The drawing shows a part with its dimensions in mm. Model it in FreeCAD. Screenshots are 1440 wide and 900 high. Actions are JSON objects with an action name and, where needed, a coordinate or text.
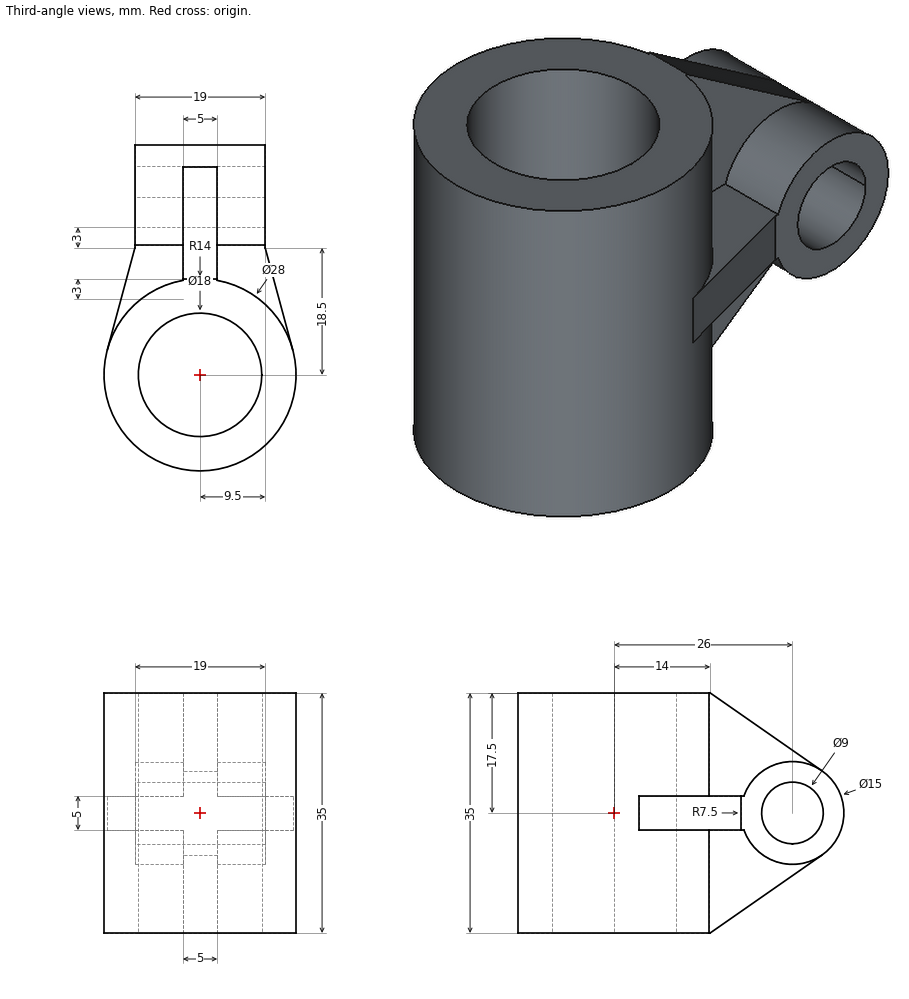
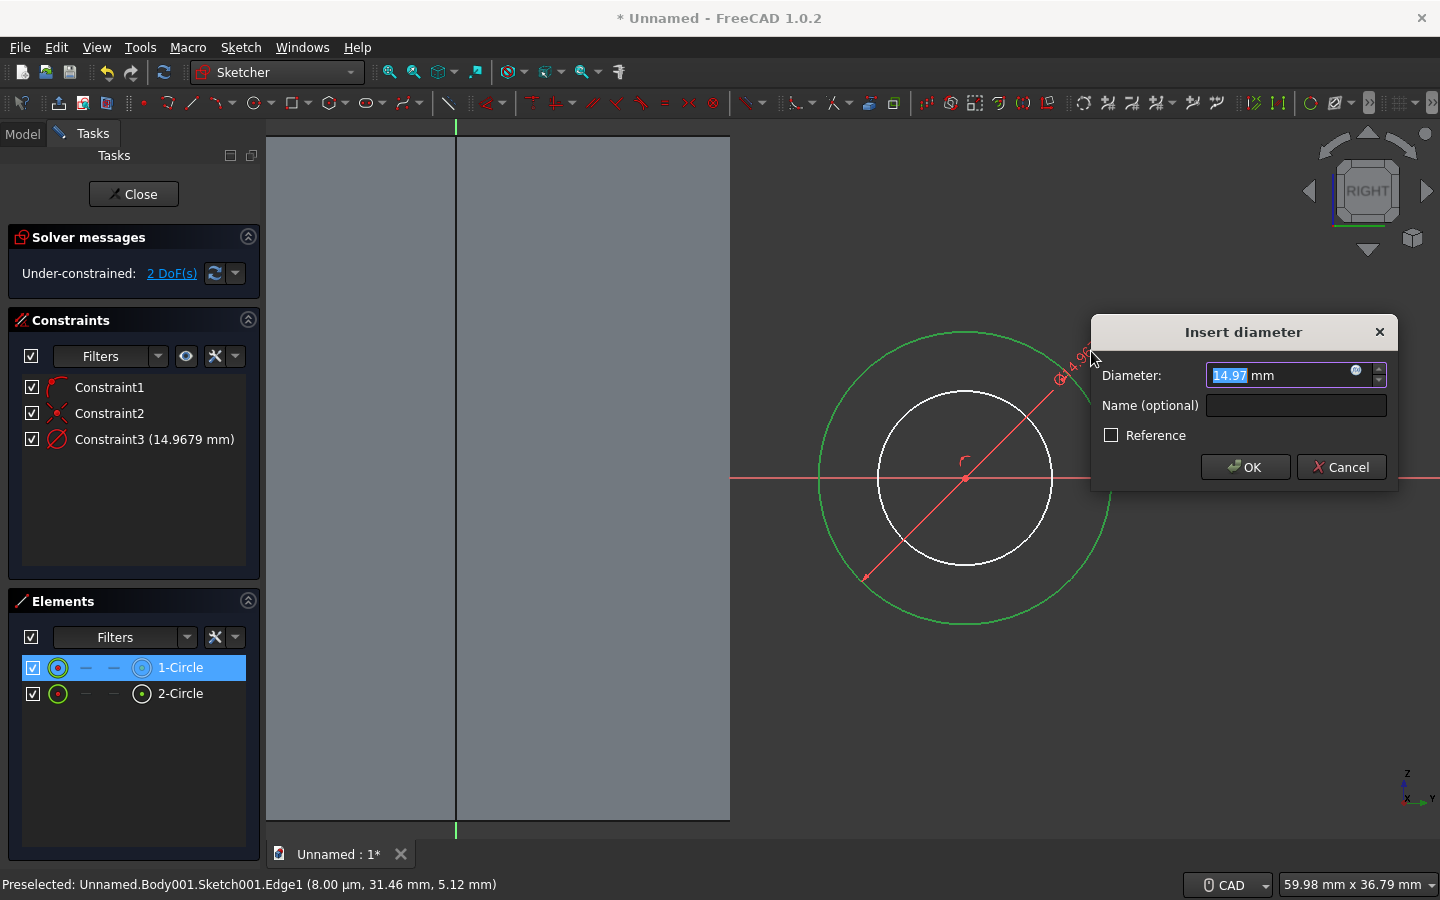
{"action": "type", "text": "15"}
{"action": "key", "text": "Return"}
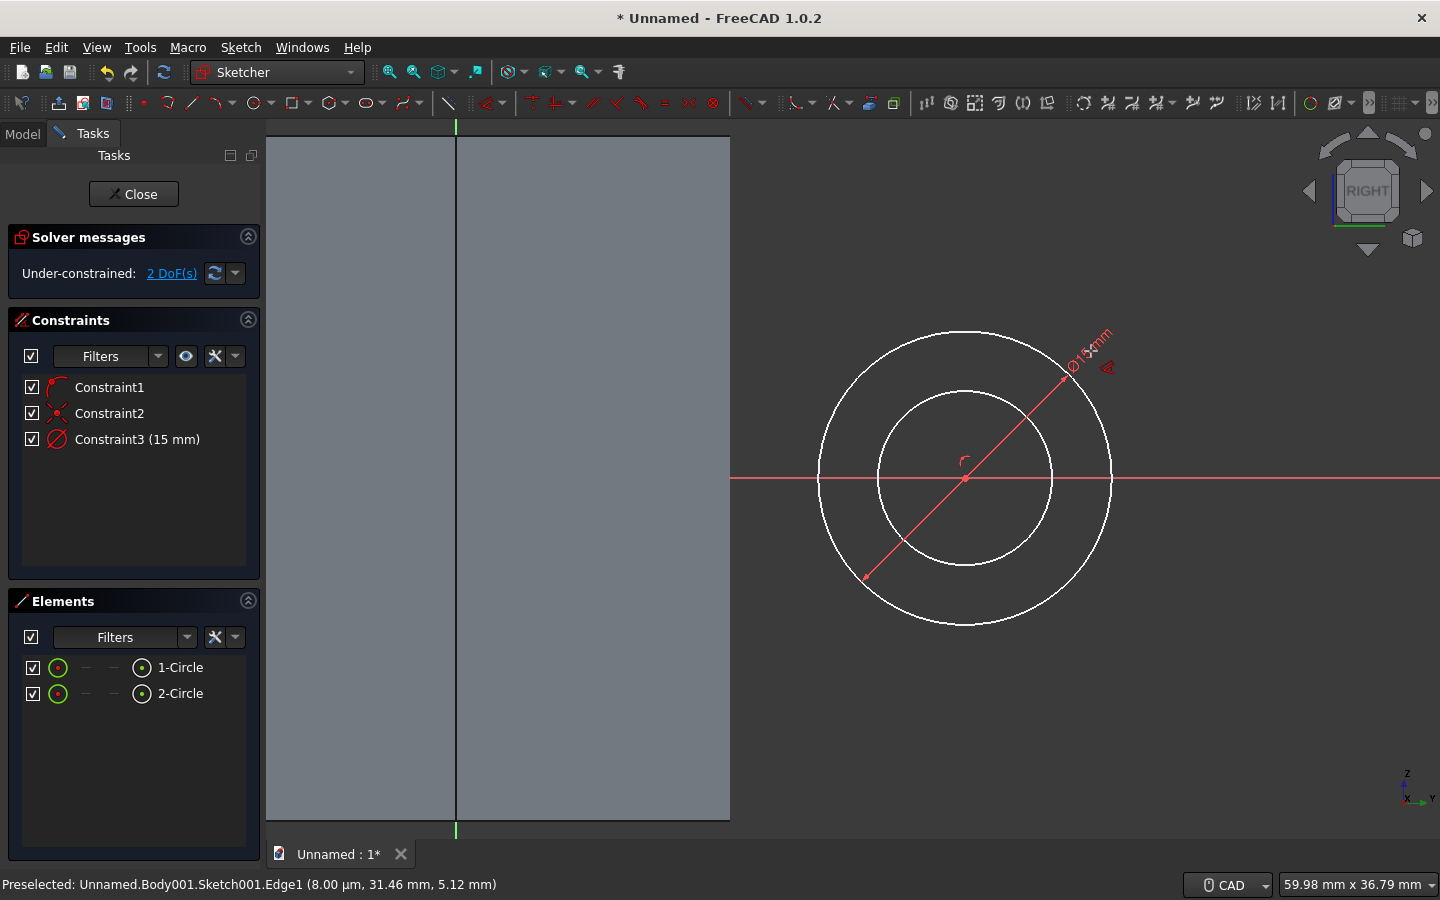
{"action": "left_click", "coordinate": [1026, 416]}
{"action": "left_click", "coordinate": [1048, 393]}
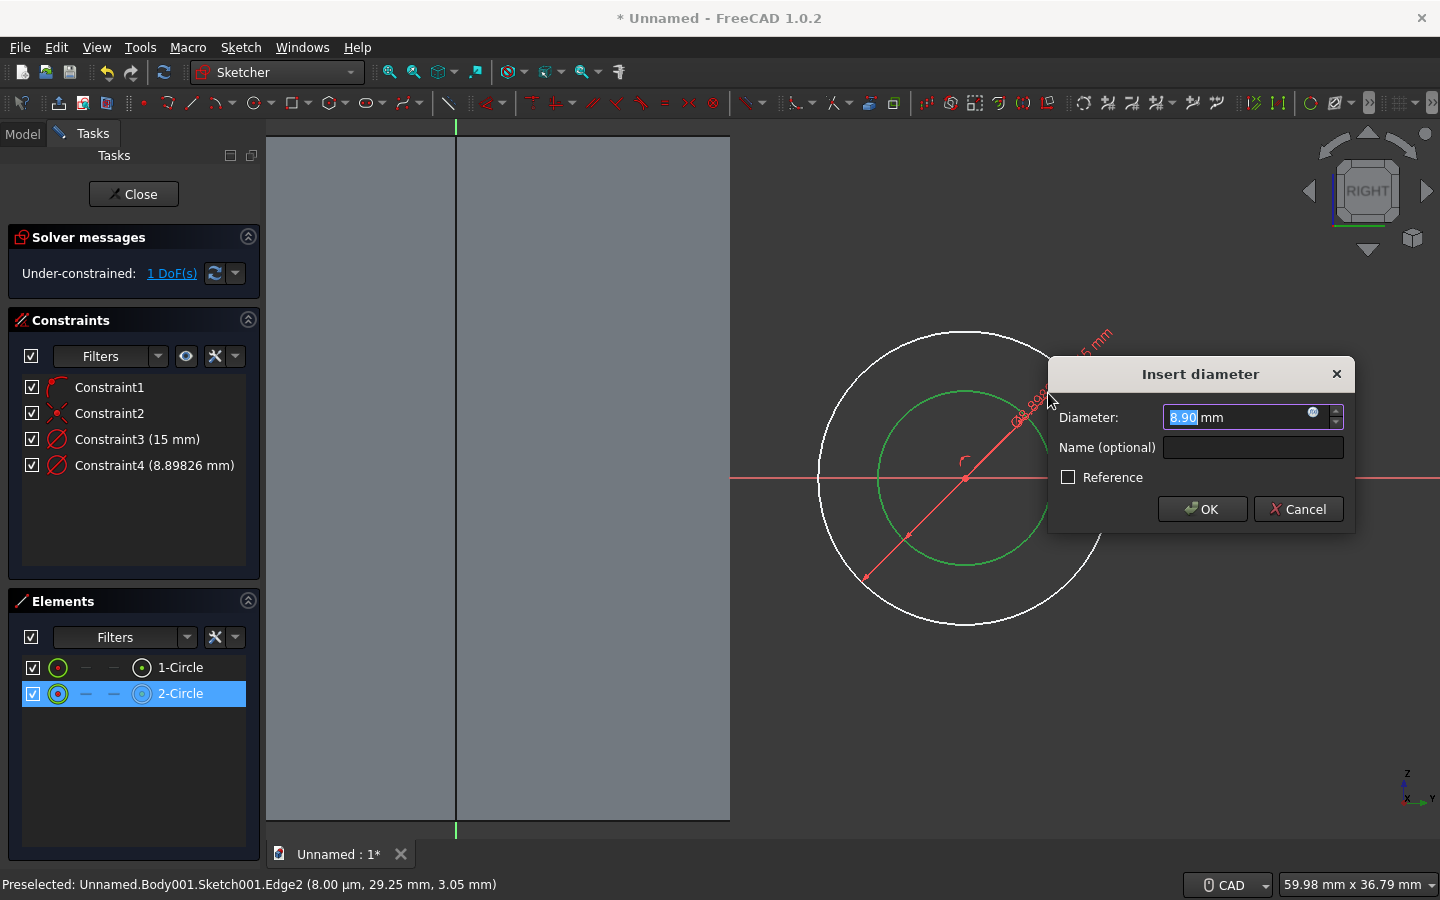
{"action": "type", "text": "9"}
{"action": "key", "text": "Return"}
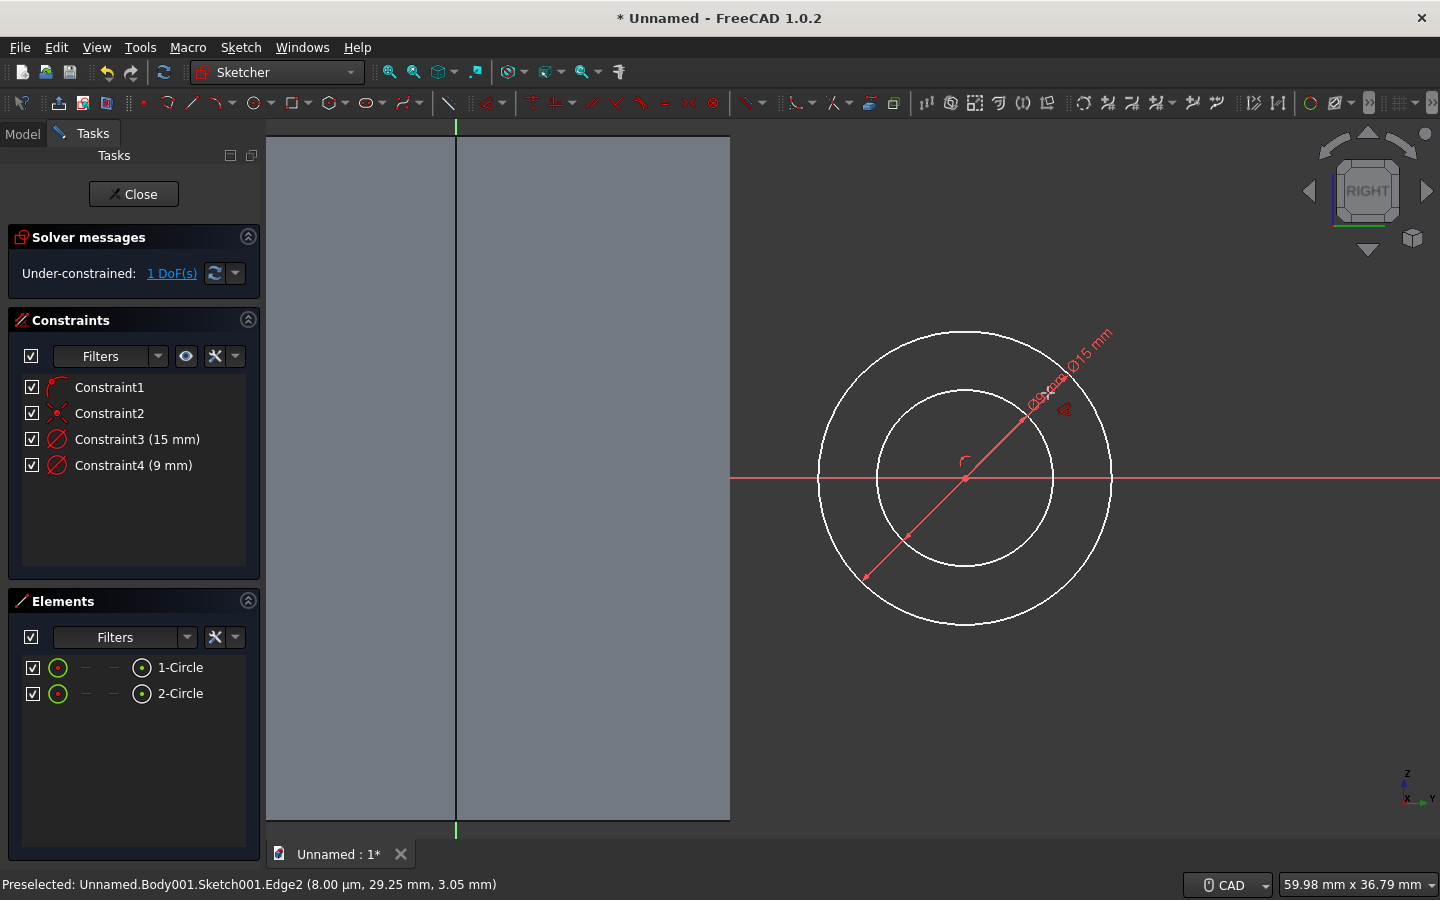
{"action": "left_click", "coordinate": [965, 478]}
{"action": "left_click", "coordinate": [710, 512]}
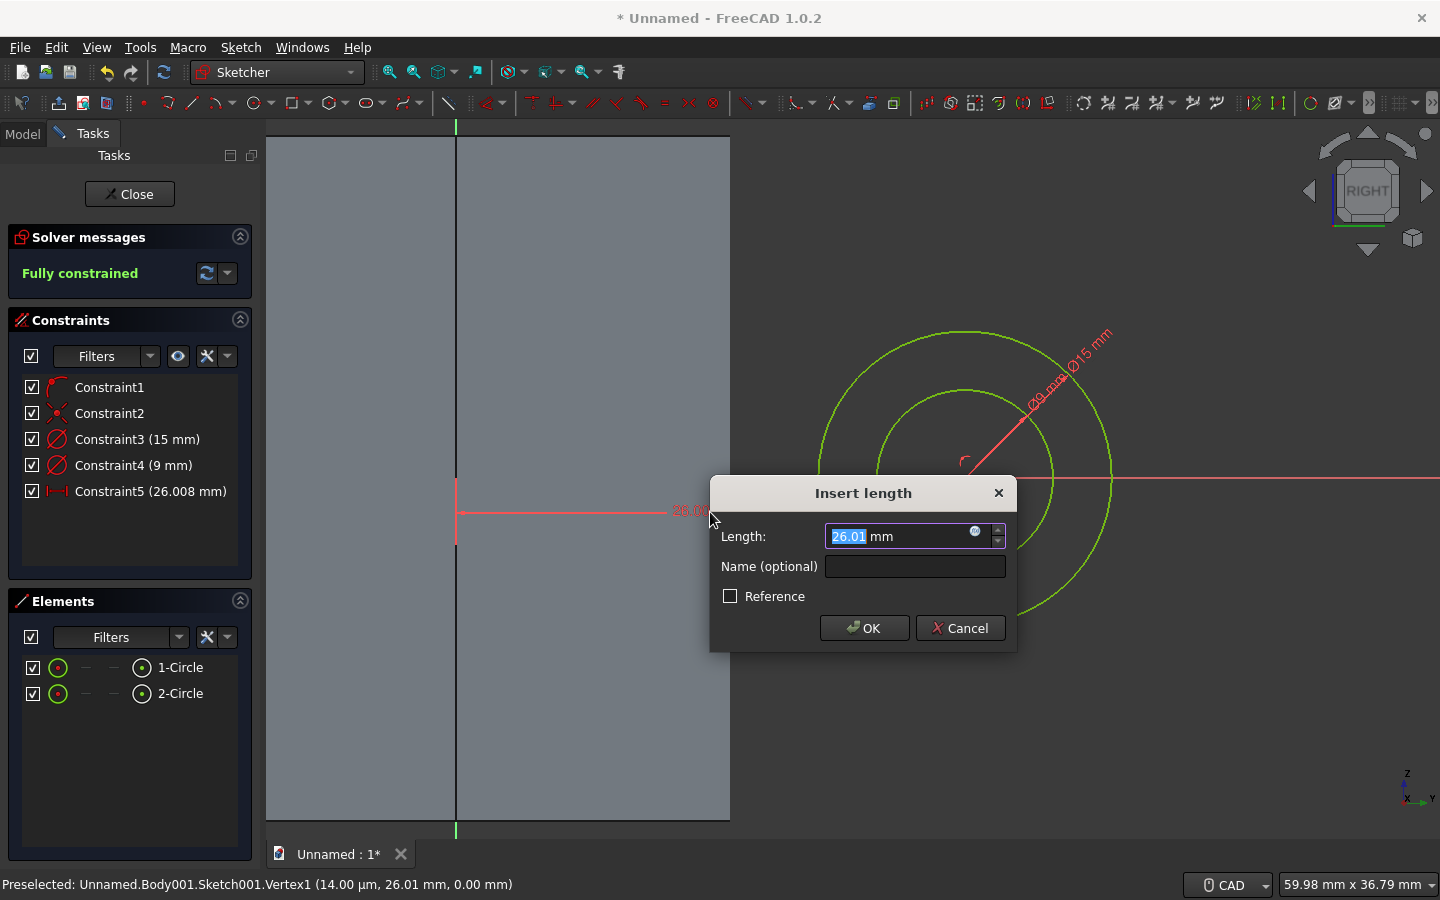
{"action": "type", "text": "26"}
{"action": "key", "text": "Return"}
{"action": "key", "text": "Escape"}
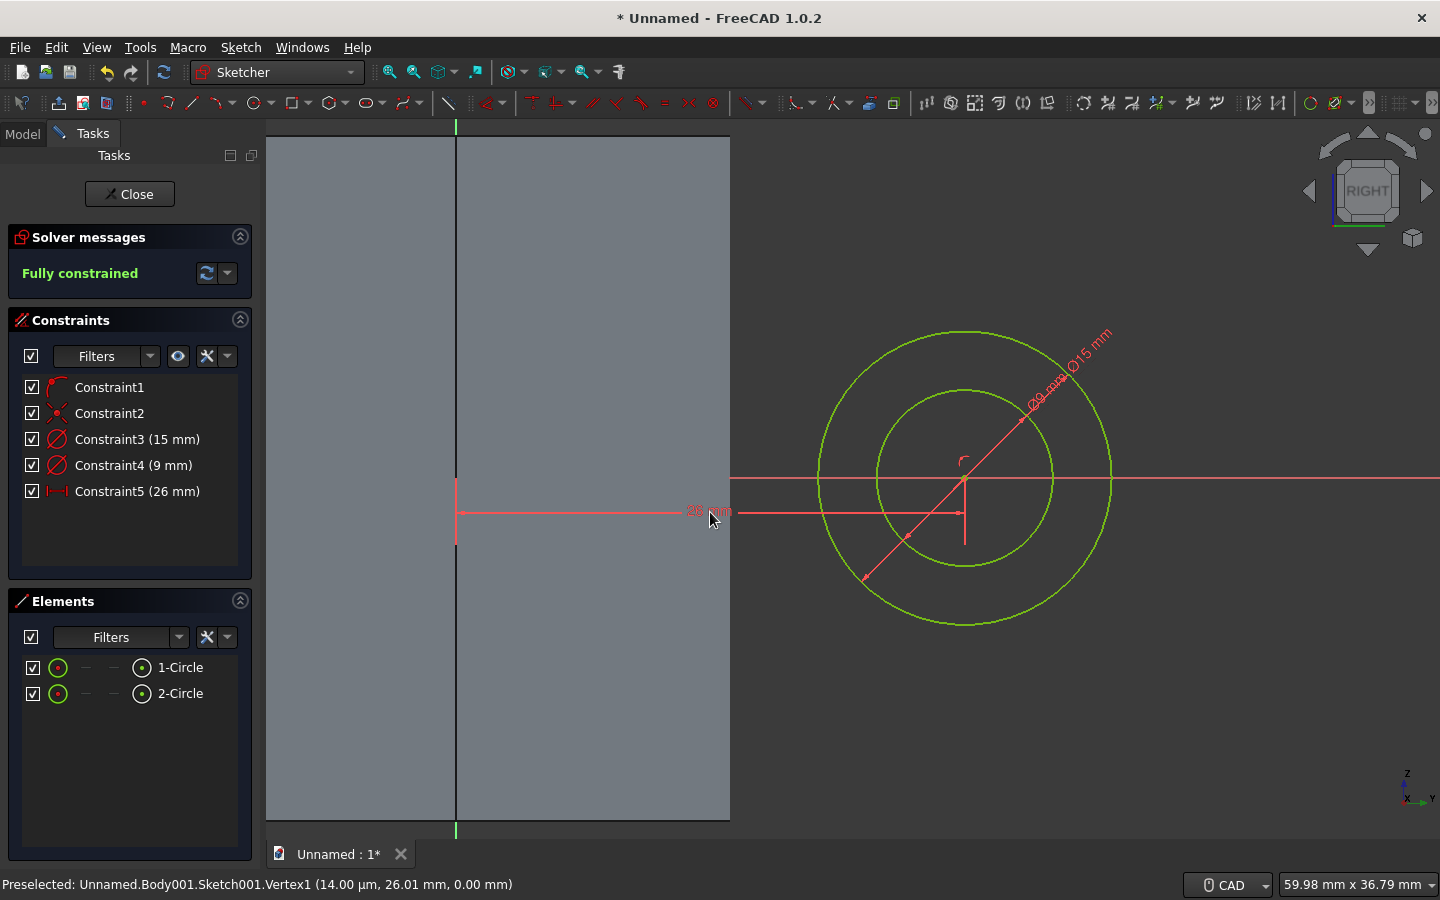
{"action": "left_click", "coordinate": [130, 194]}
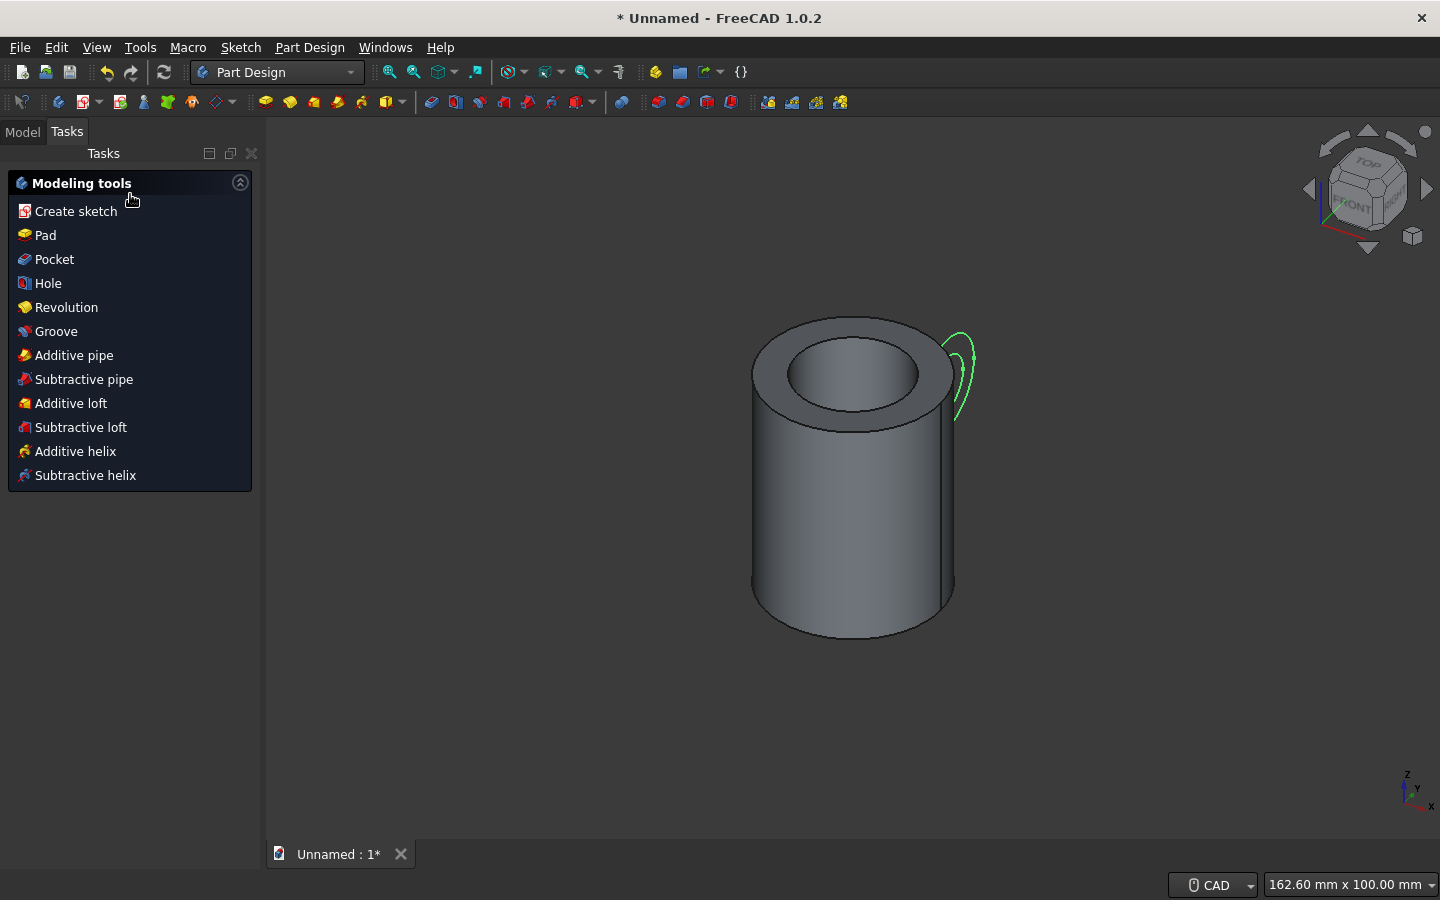
{"action": "left_click", "coordinate": [266, 102]}